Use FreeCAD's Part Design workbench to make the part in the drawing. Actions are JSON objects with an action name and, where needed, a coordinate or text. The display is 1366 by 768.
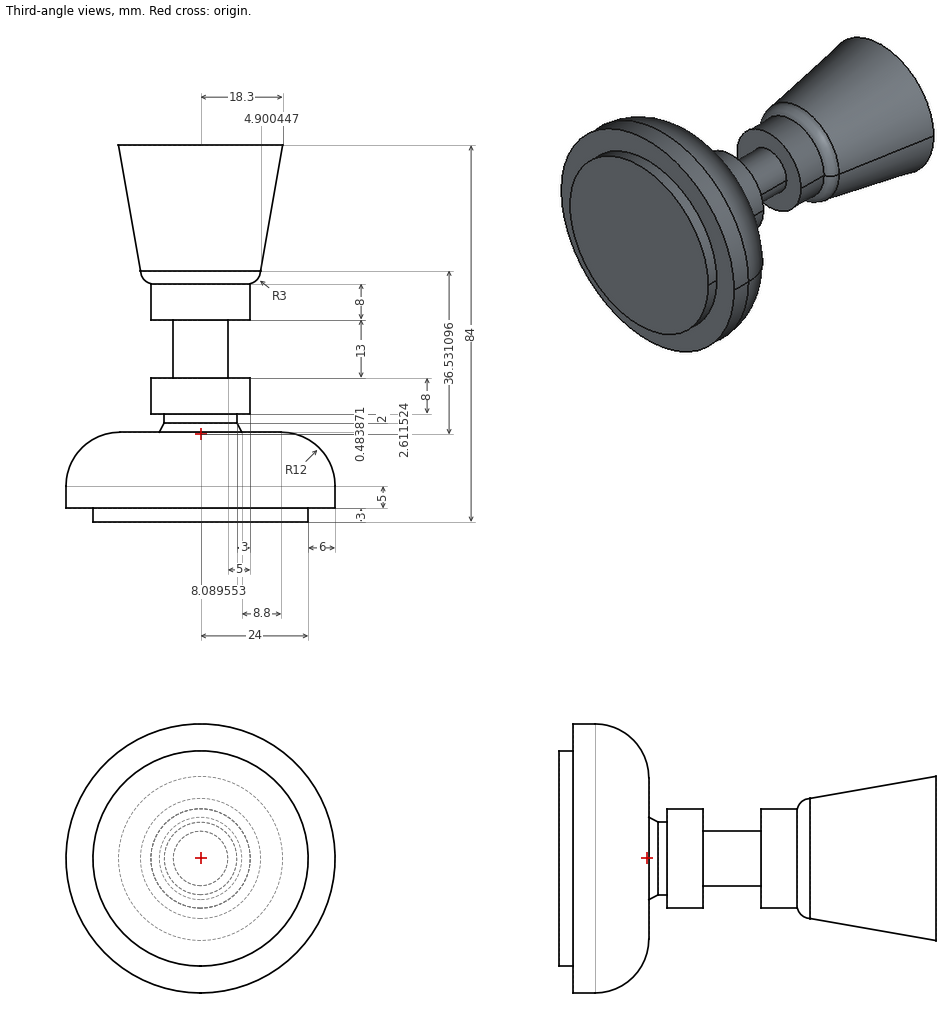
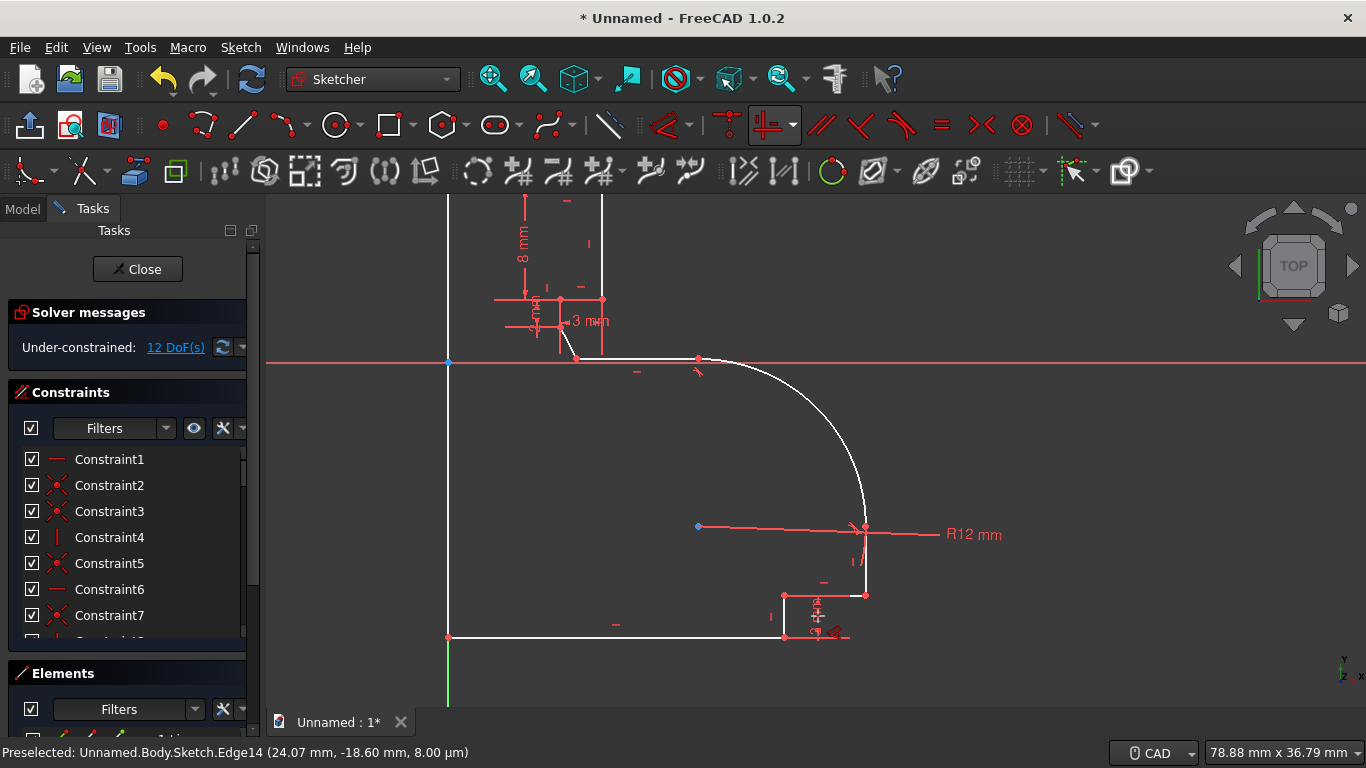
{"action": "left_click", "coordinate": [809, 596]}
{"action": "left_click", "coordinate": [825, 562]}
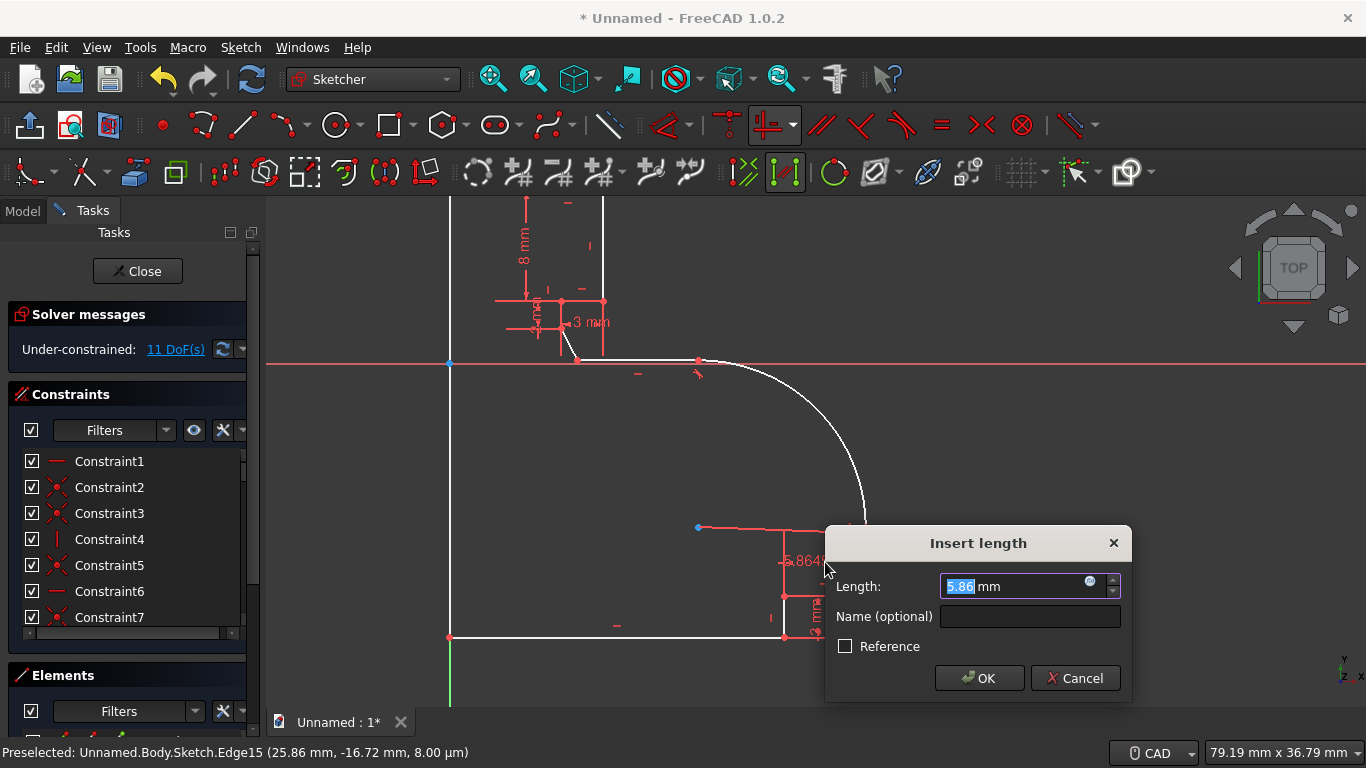
{"action": "type", "text": "6"}
{"action": "key", "text": "Return"}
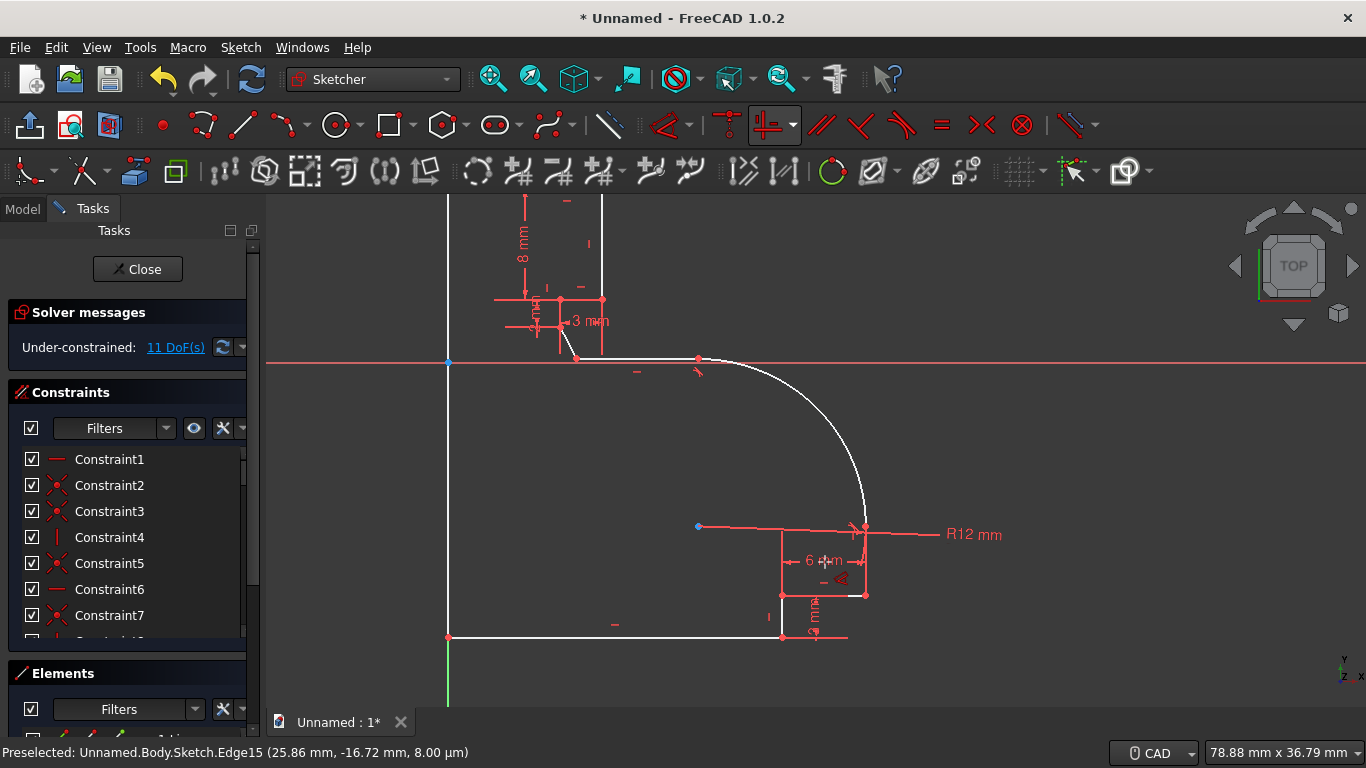
{"action": "left_click", "coordinate": [866, 575]}
{"action": "left_click", "coordinate": [900, 561]}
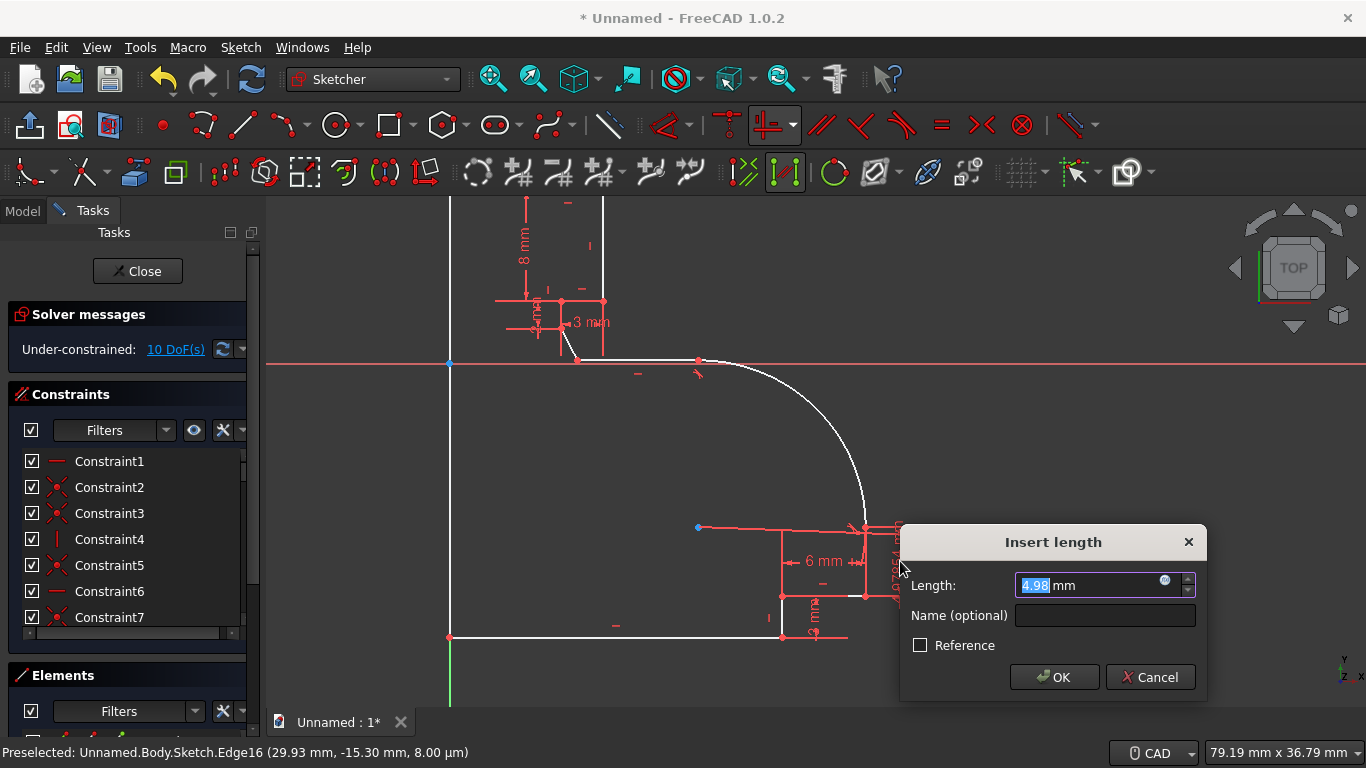
{"action": "type", "text": "5"}
{"action": "key", "text": "Return"}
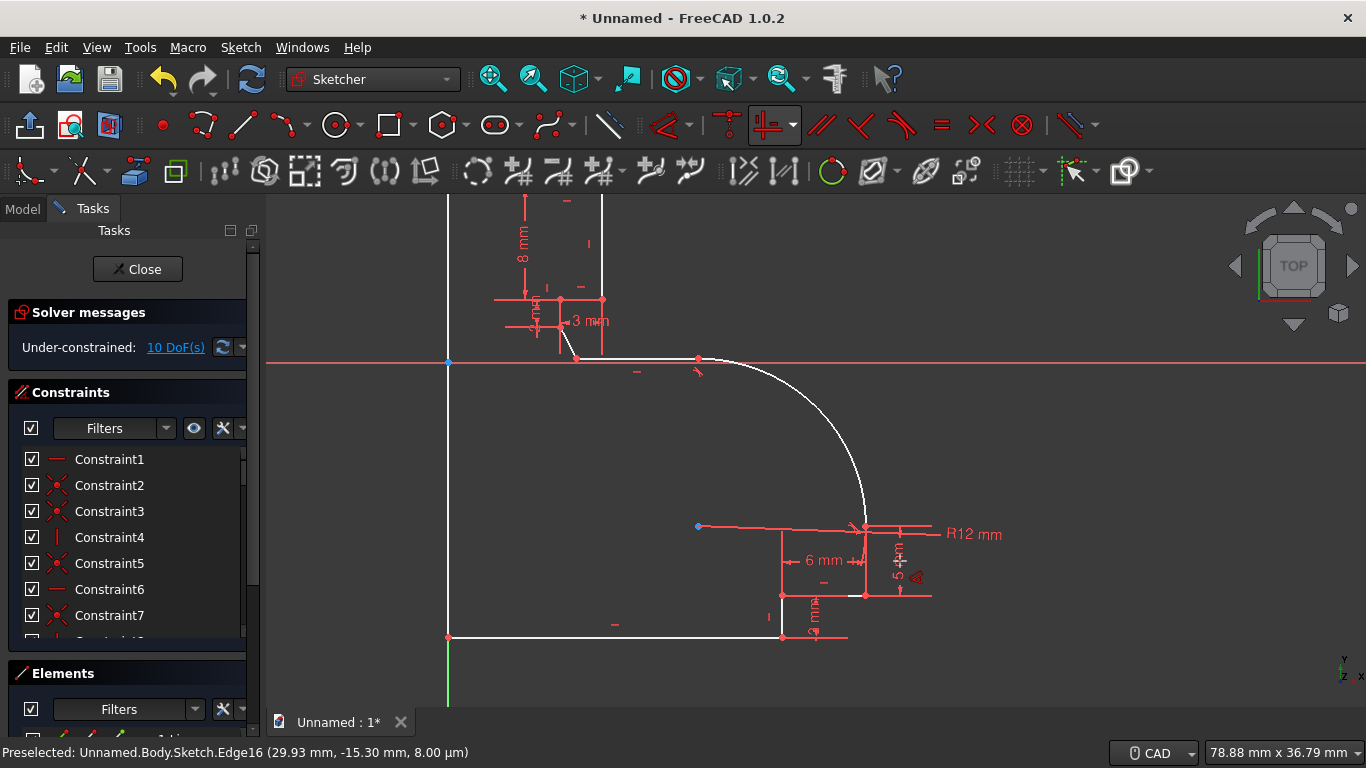
{"action": "scroll", "coordinate": [786, 624], "scroll_direction": "down", "scroll_amount": 6}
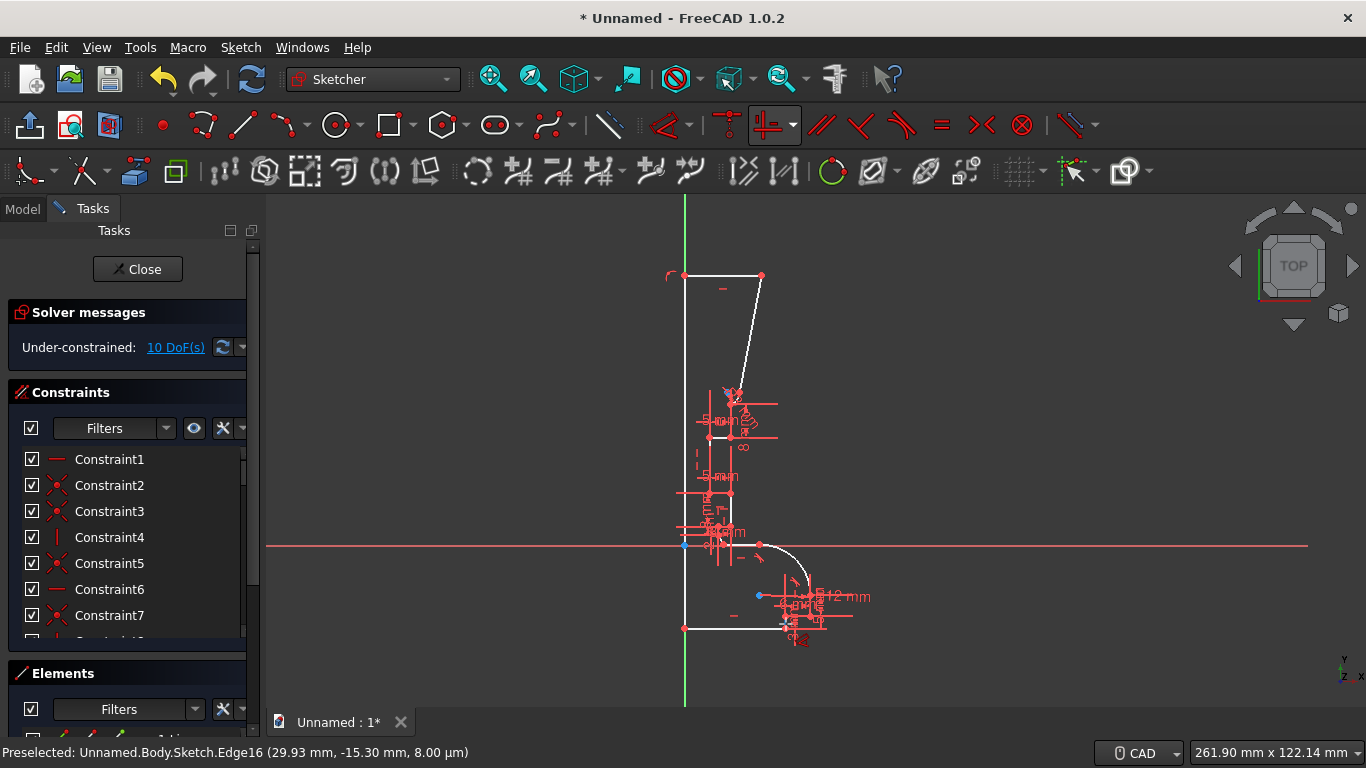
{"action": "left_click", "coordinate": [710, 477]}
{"action": "left_click", "coordinate": [652, 453]}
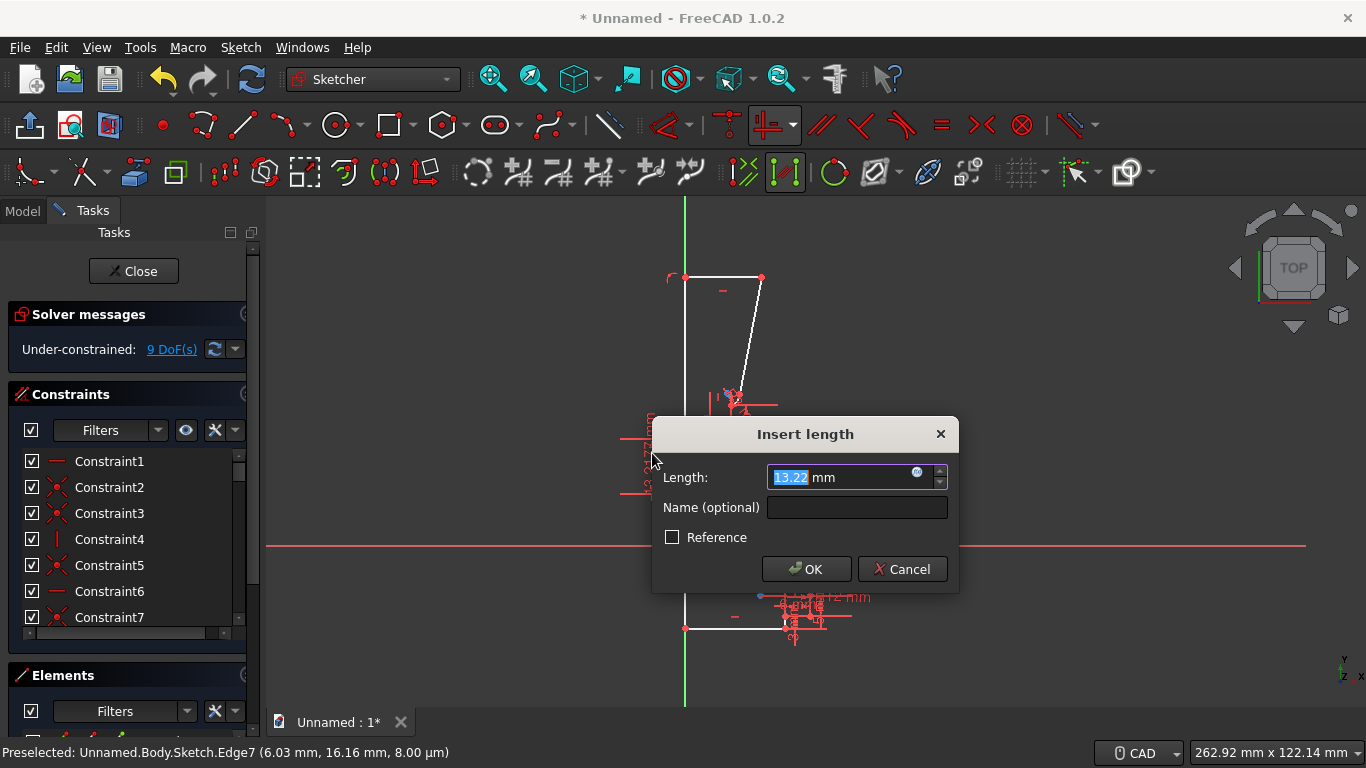
{"action": "type", "text": "13"}
{"action": "key", "text": "Return"}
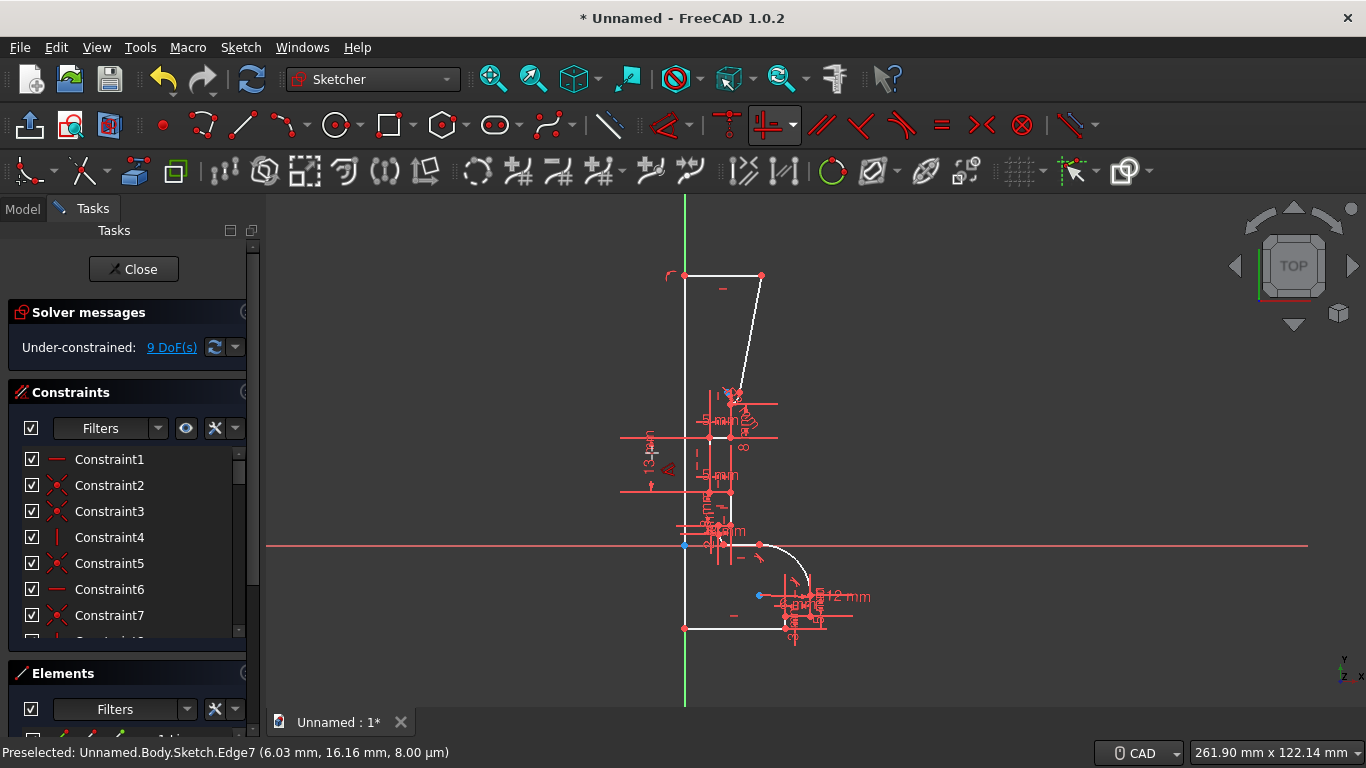
{"action": "left_click", "coordinate": [685, 382]}
{"action": "left_click", "coordinate": [651, 371]}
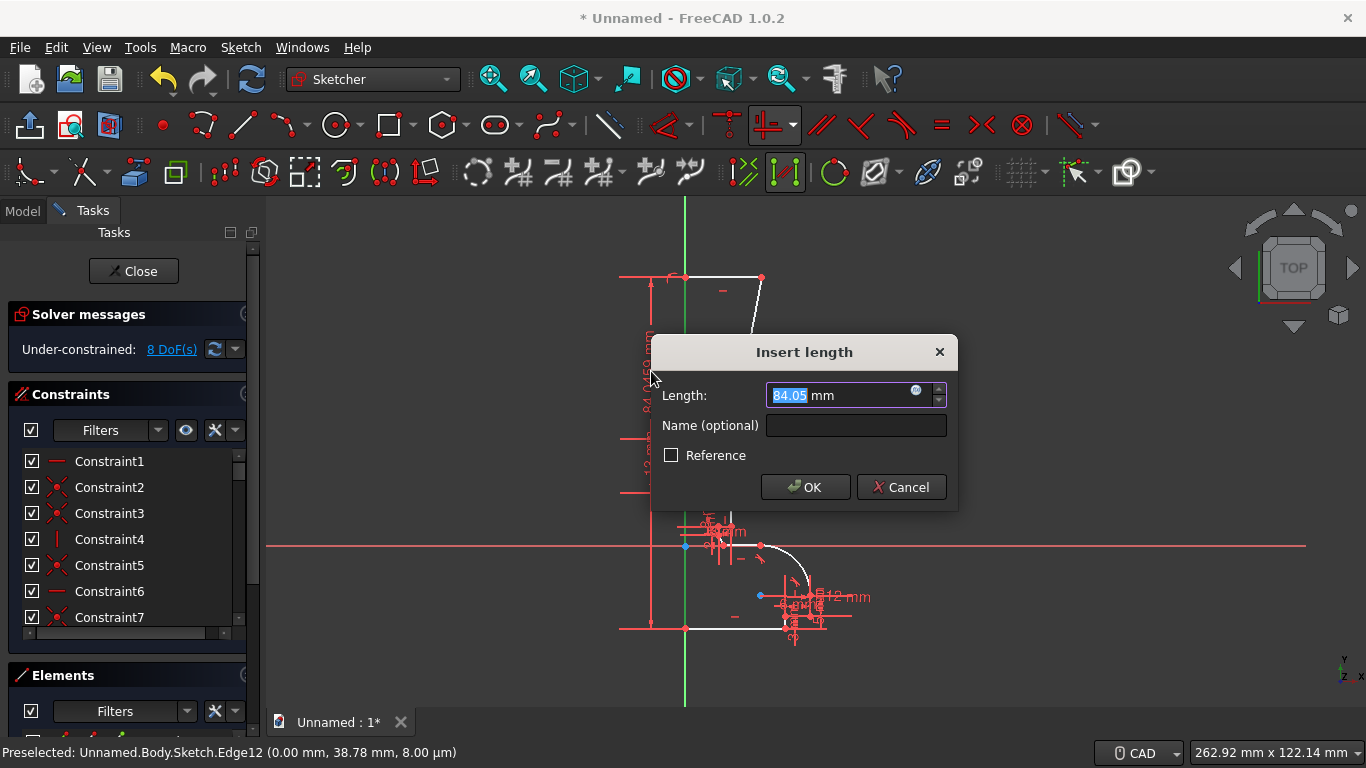
{"action": "type", "text": "84"}
{"action": "key", "text": "Return"}